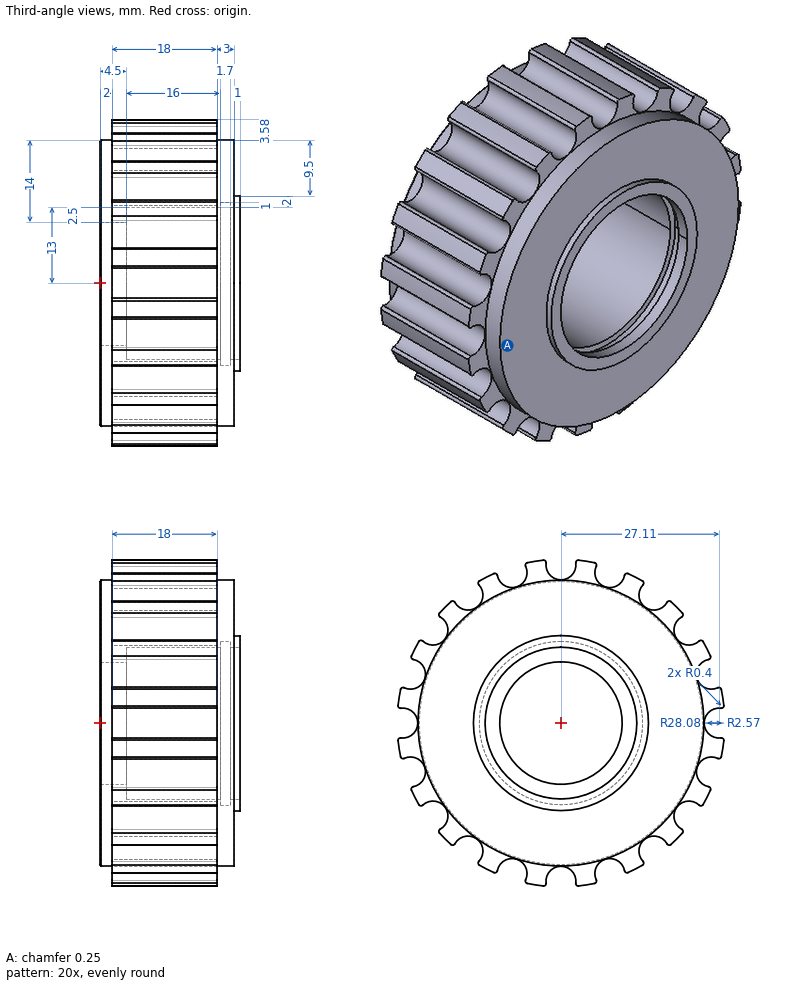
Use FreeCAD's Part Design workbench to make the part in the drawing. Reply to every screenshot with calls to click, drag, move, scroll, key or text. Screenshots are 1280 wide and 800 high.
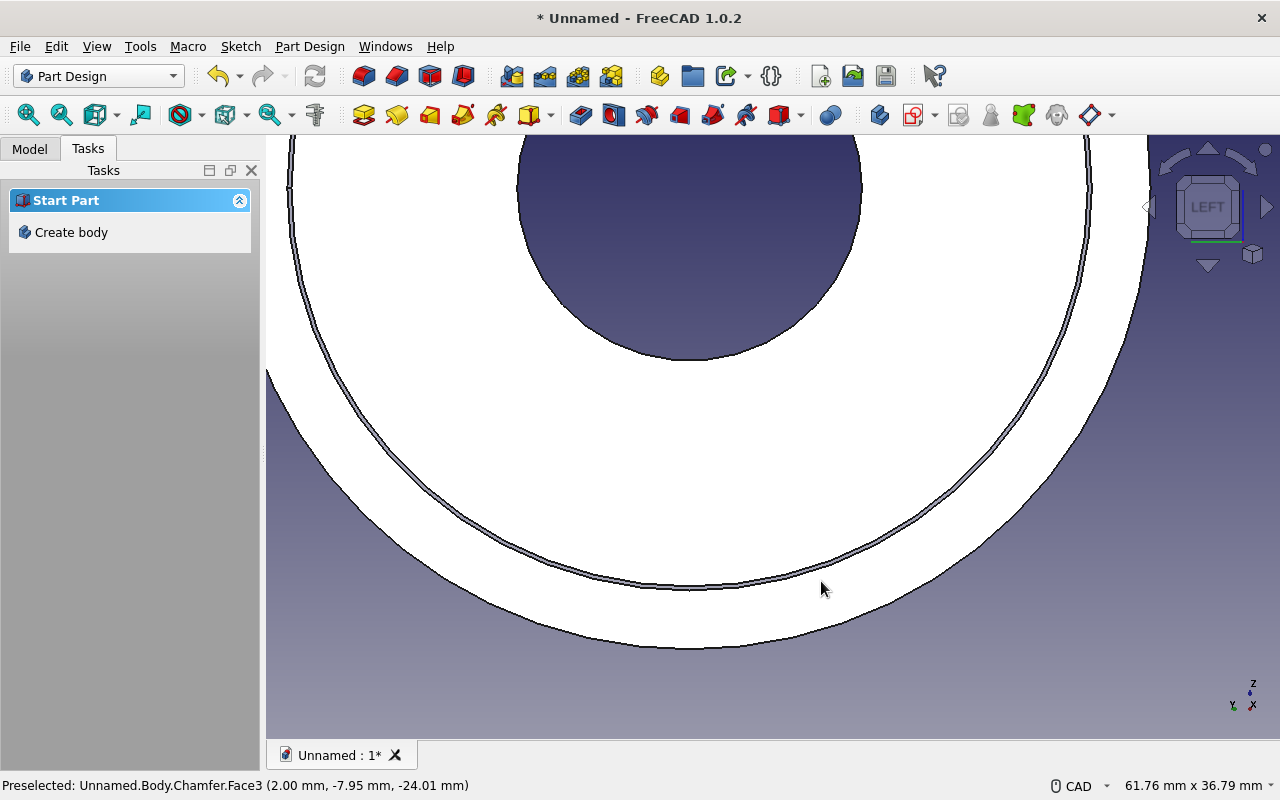
click(821, 582)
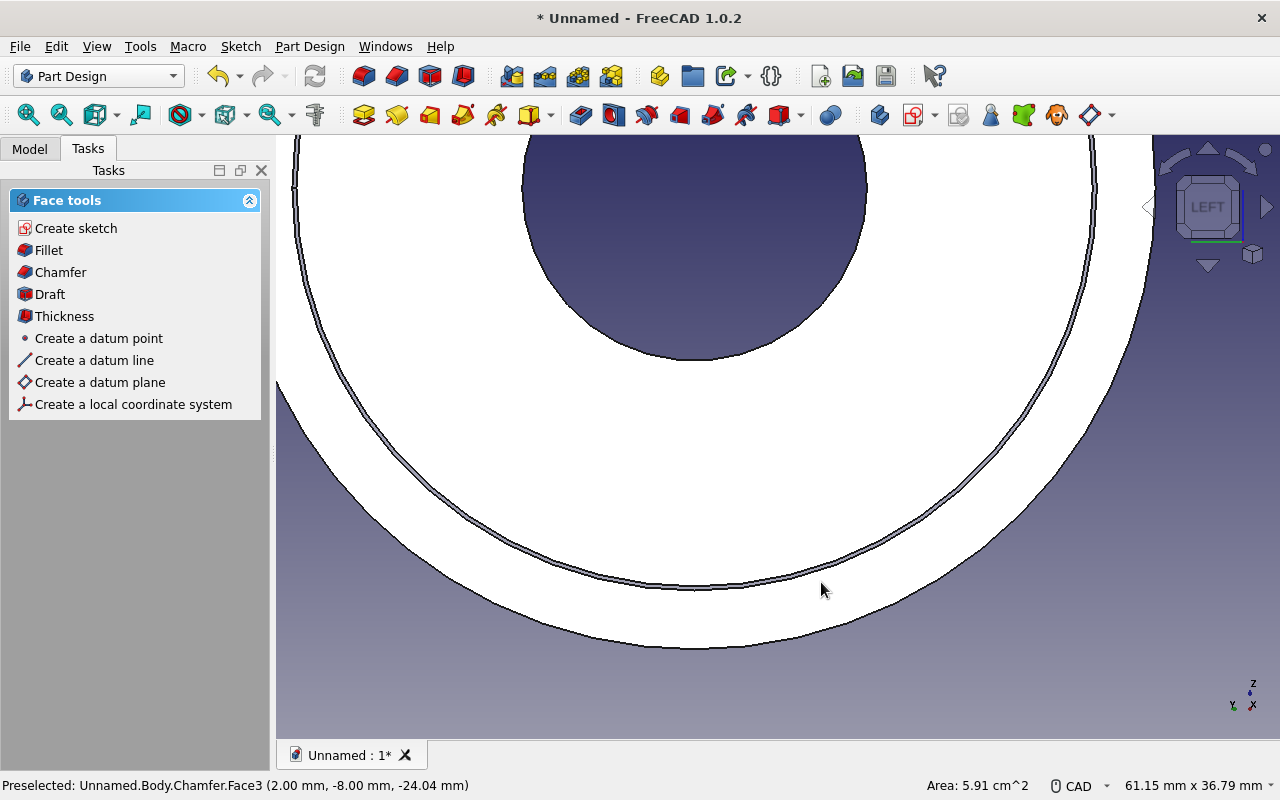
click(912, 116)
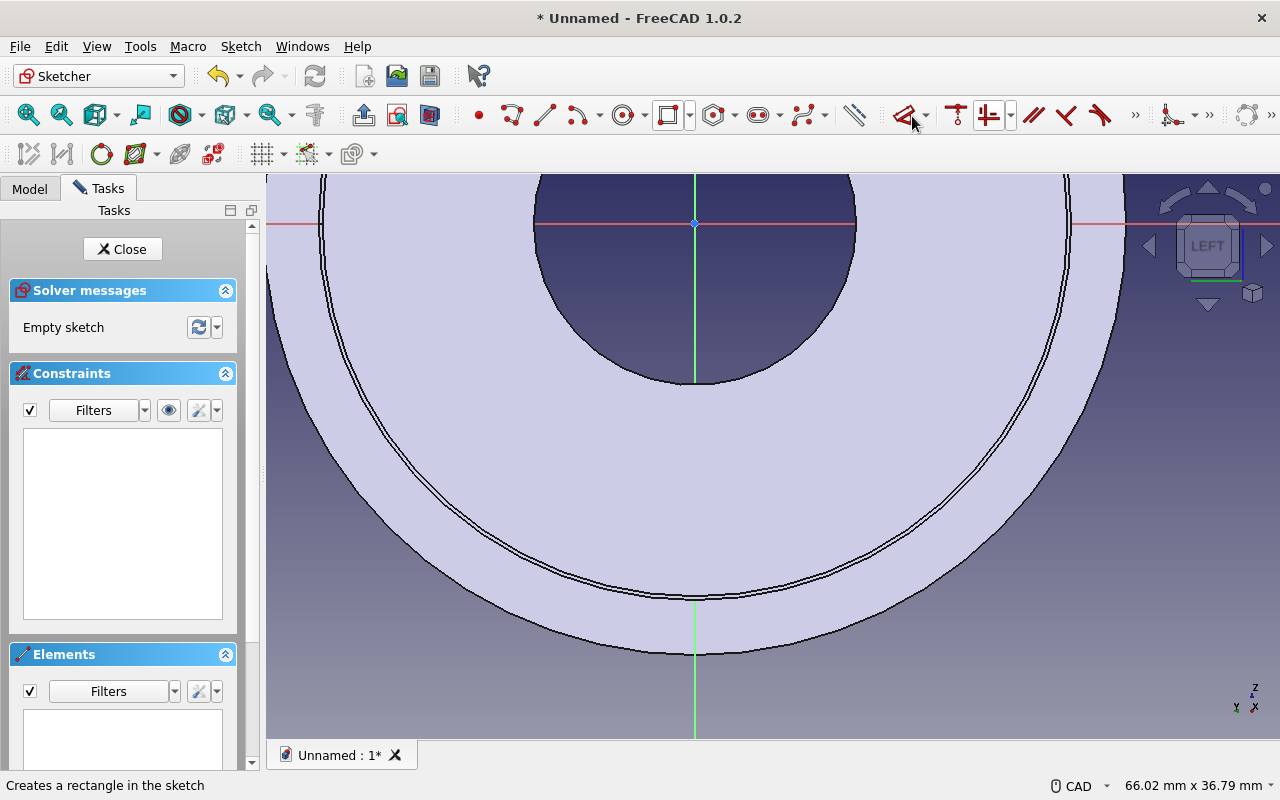
scroll(704, 456, down, 5)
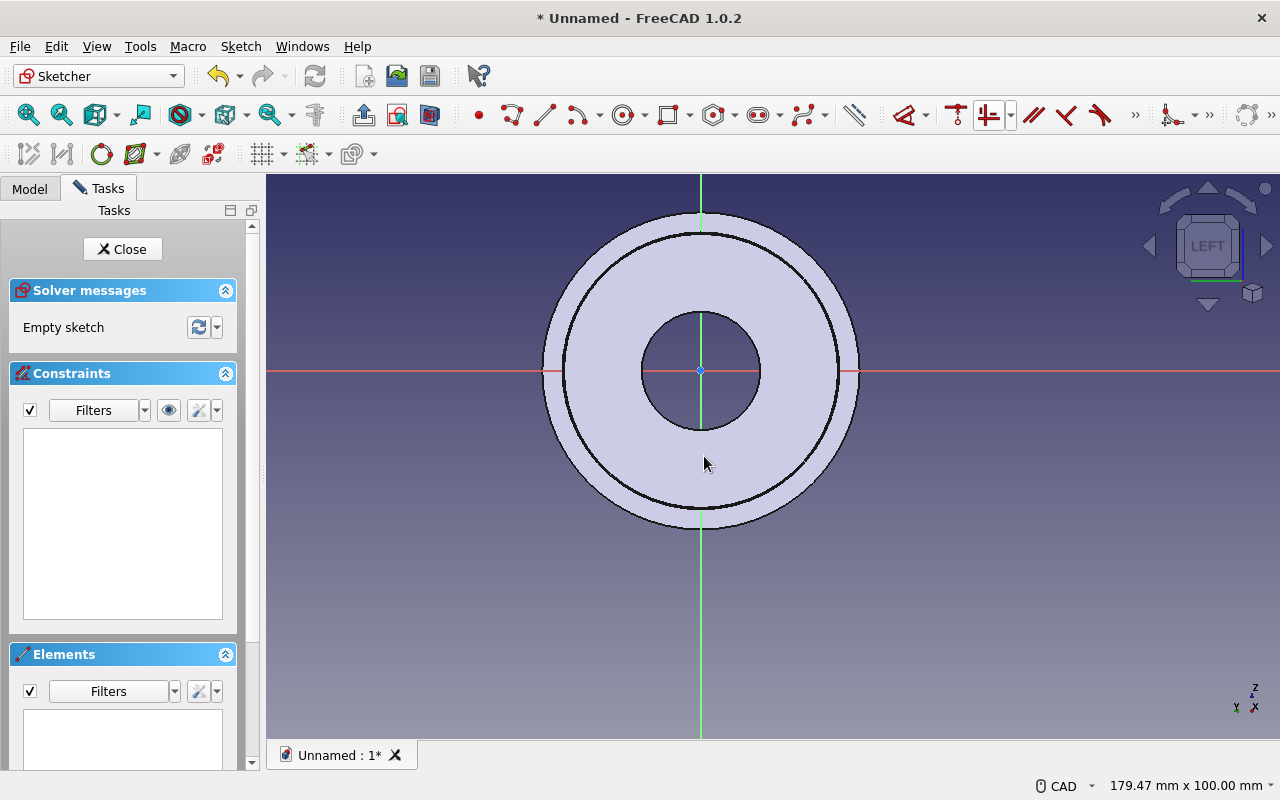
scroll(537, 362, up, 12)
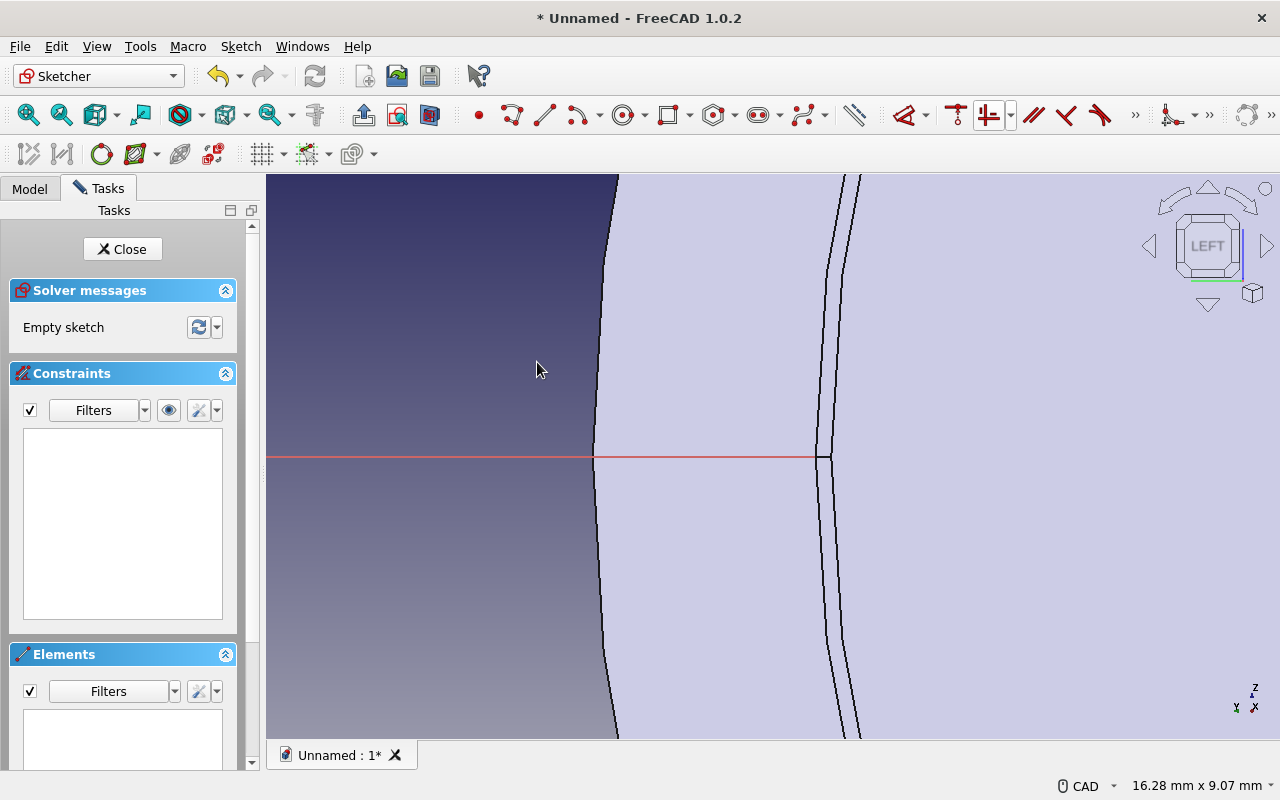
click(600, 116)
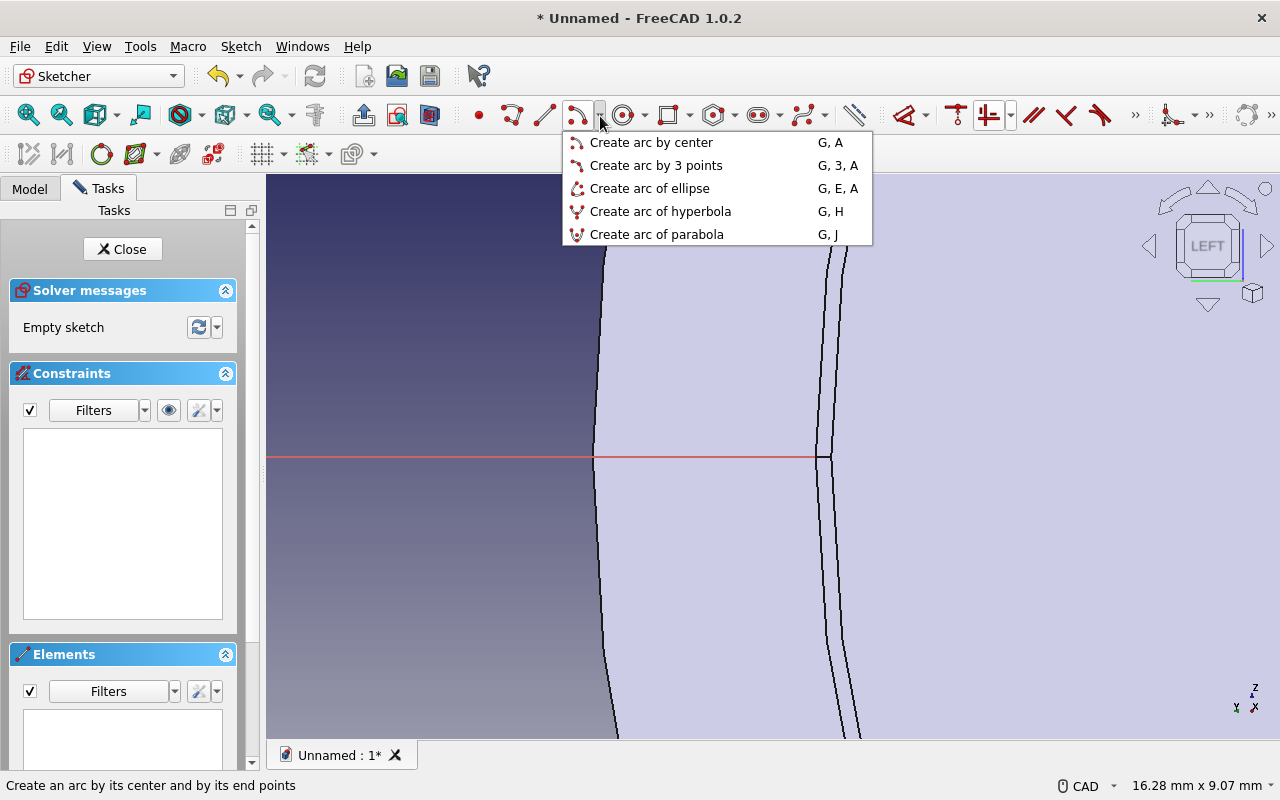
click(718, 166)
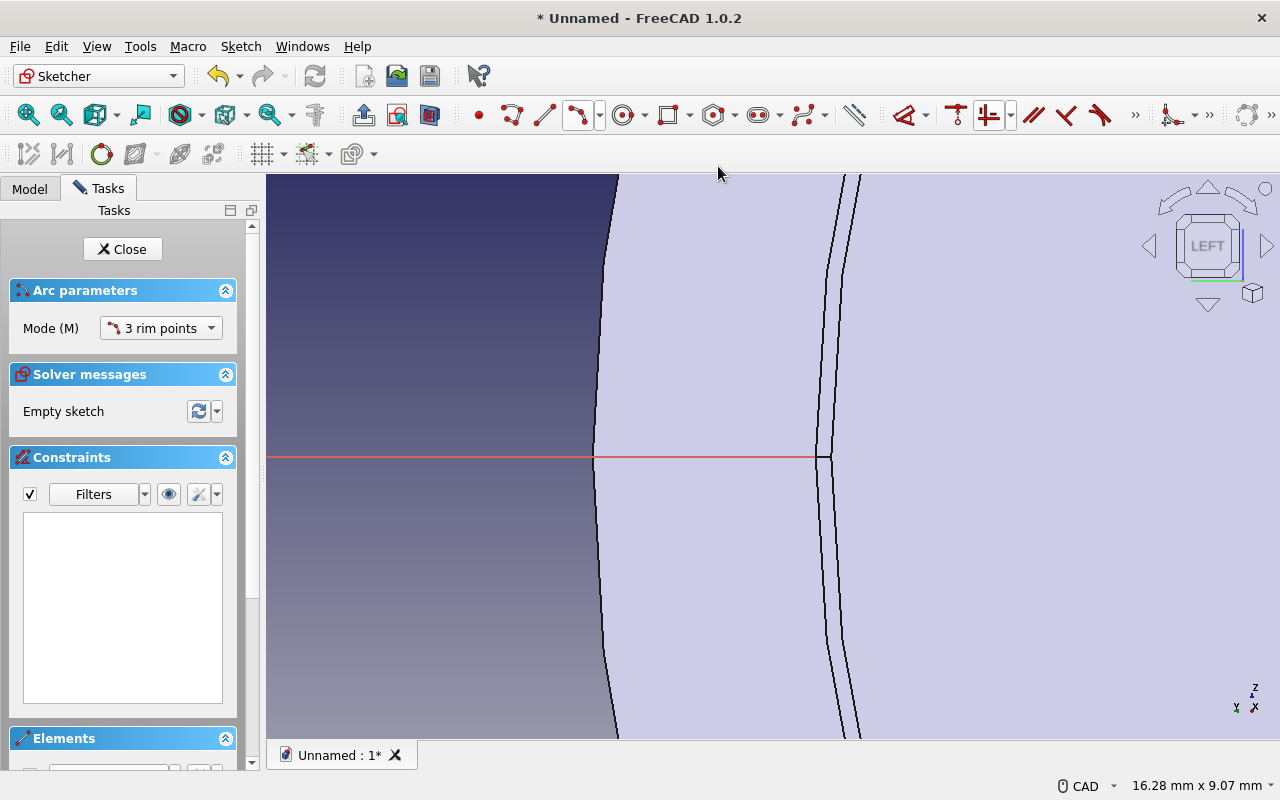
click(631, 298)
click(631, 615)
click(804, 511)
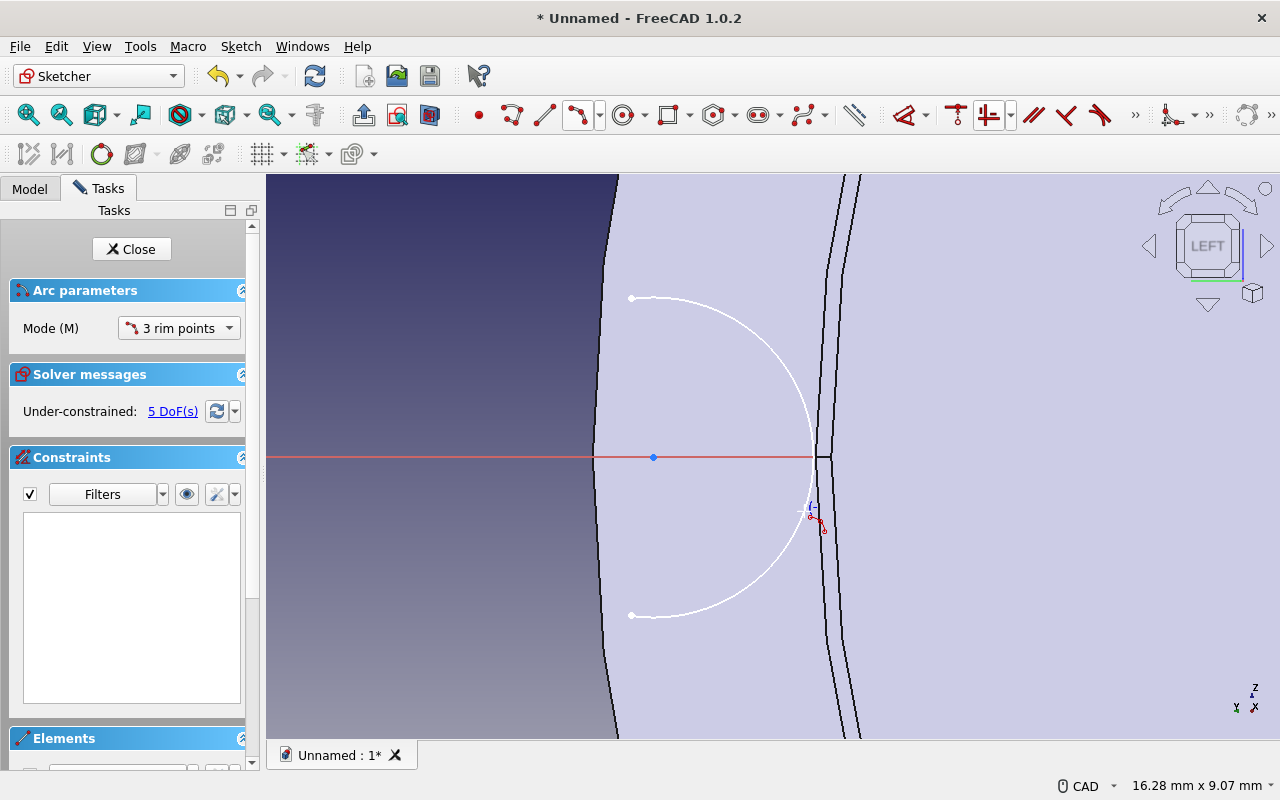
click(631, 616)
click(603, 643)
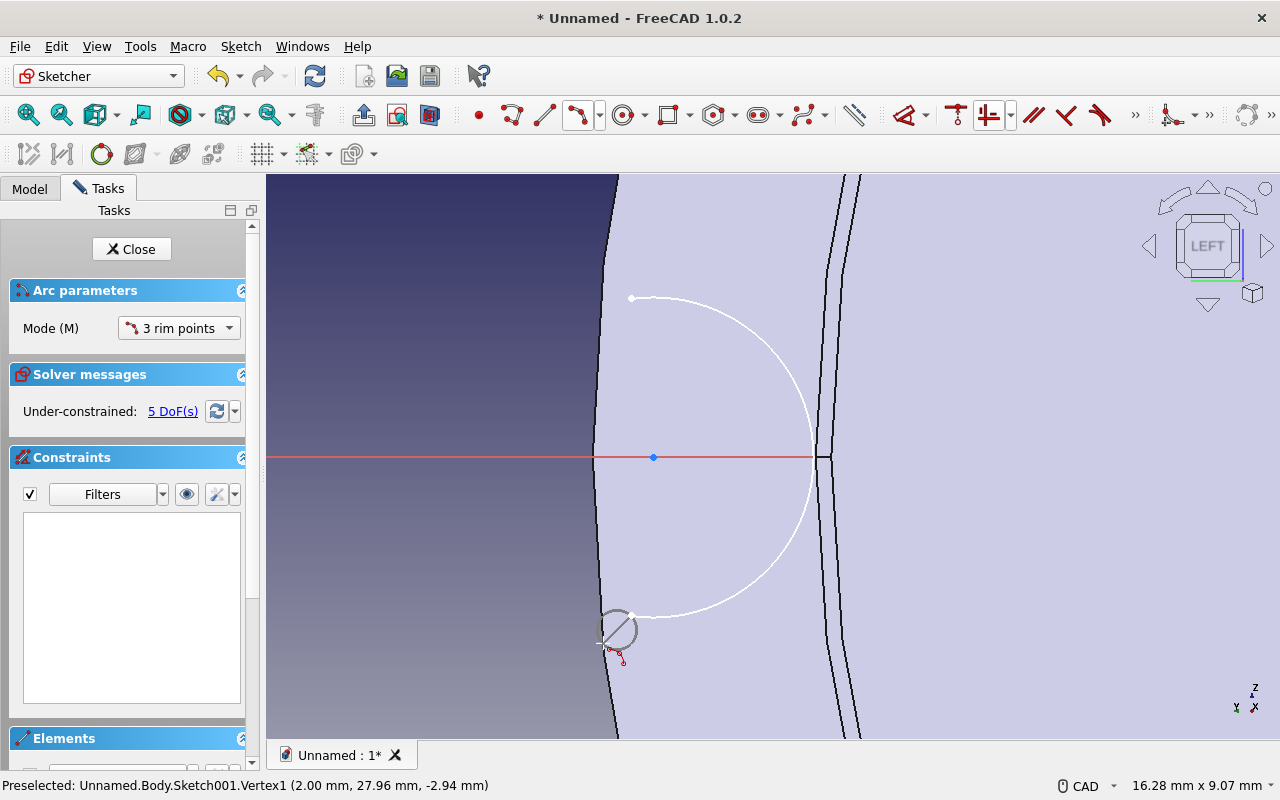
scroll(610, 622, up, 3)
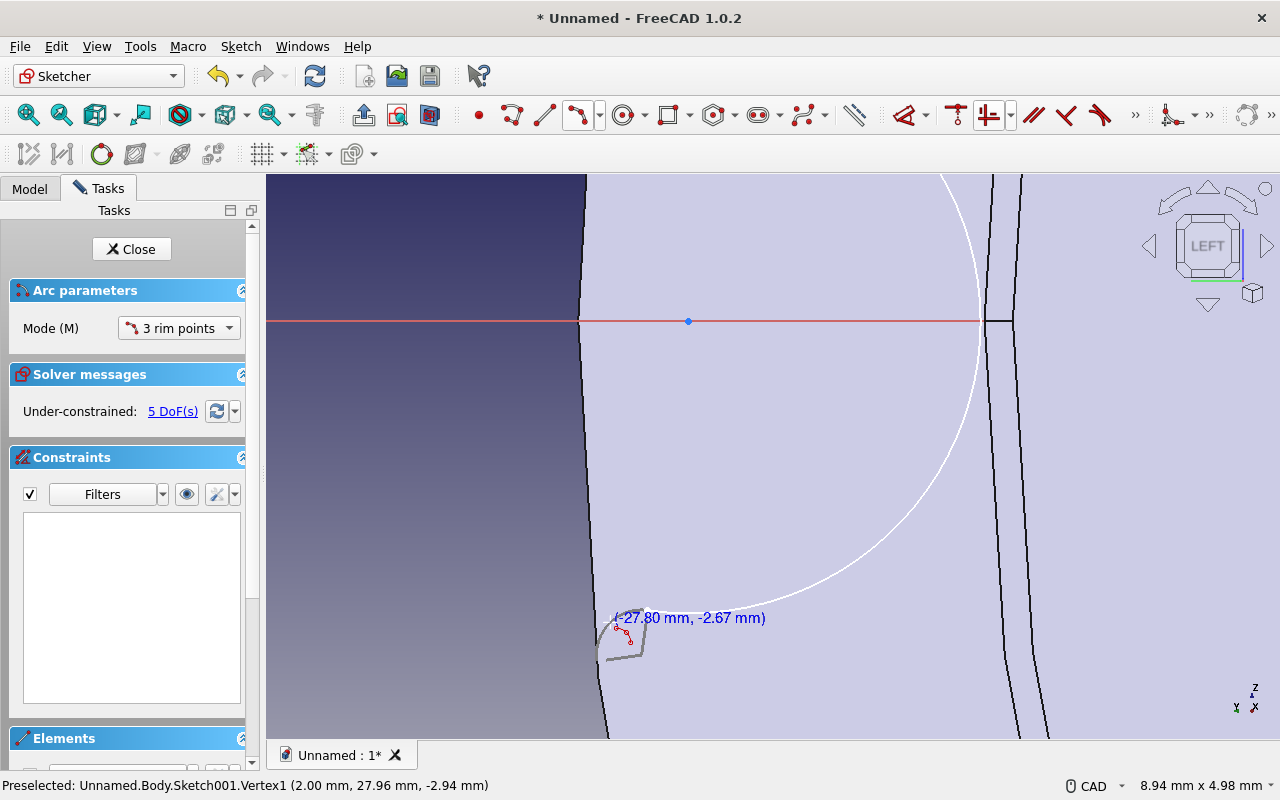
click(610, 622)